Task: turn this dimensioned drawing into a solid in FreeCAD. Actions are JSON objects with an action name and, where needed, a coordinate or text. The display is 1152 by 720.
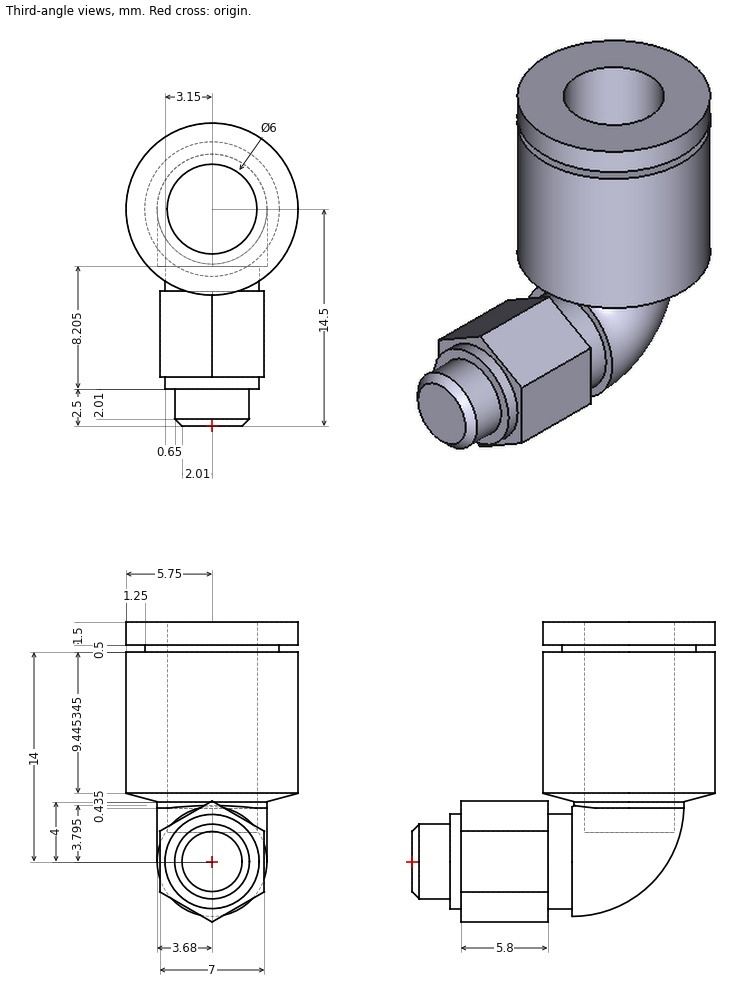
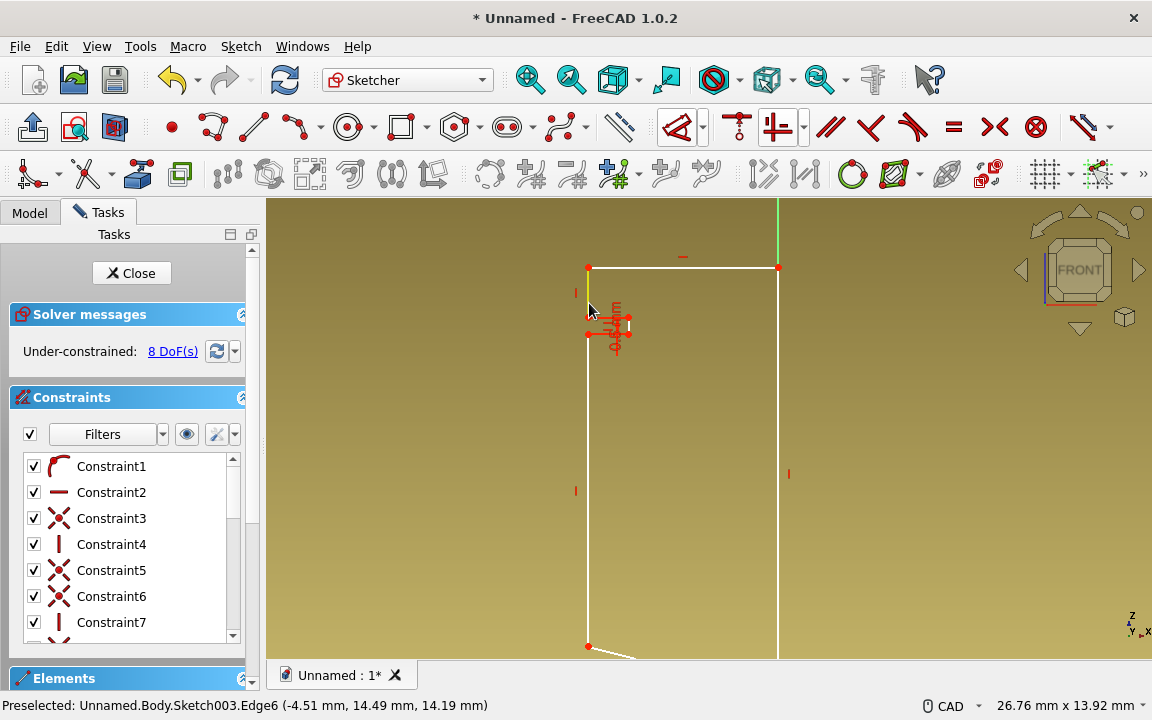
{"action": "left_click", "coordinate": [588, 303]}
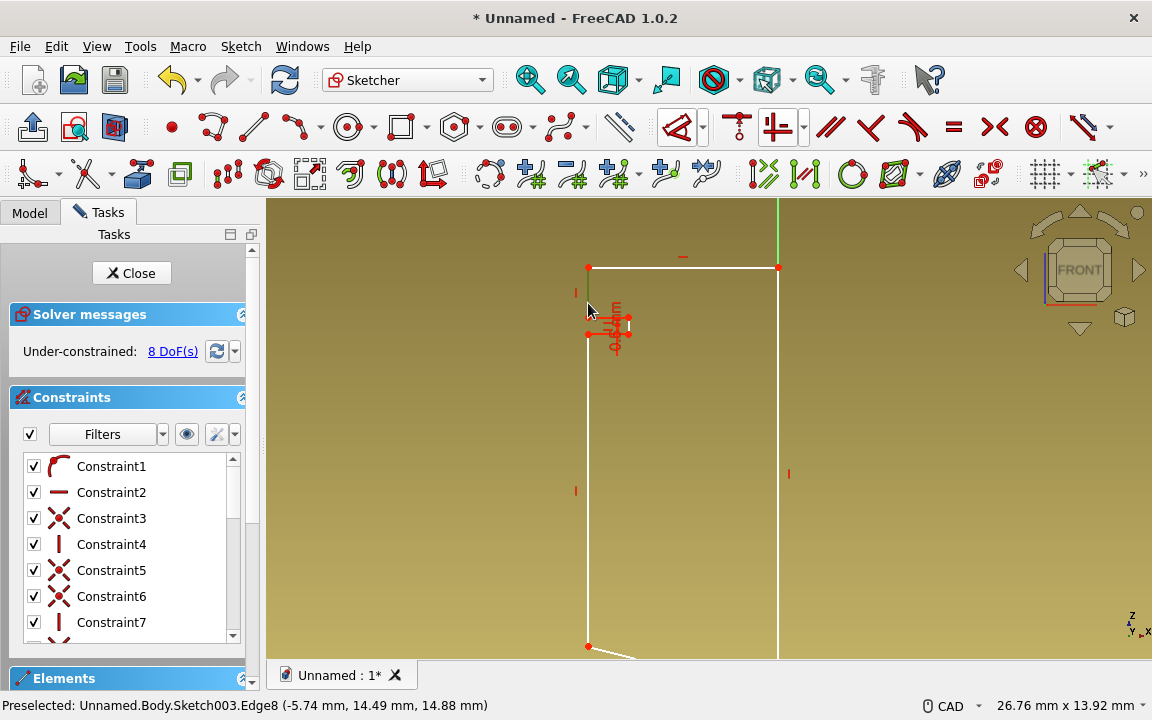
{"action": "key", "text": "i"}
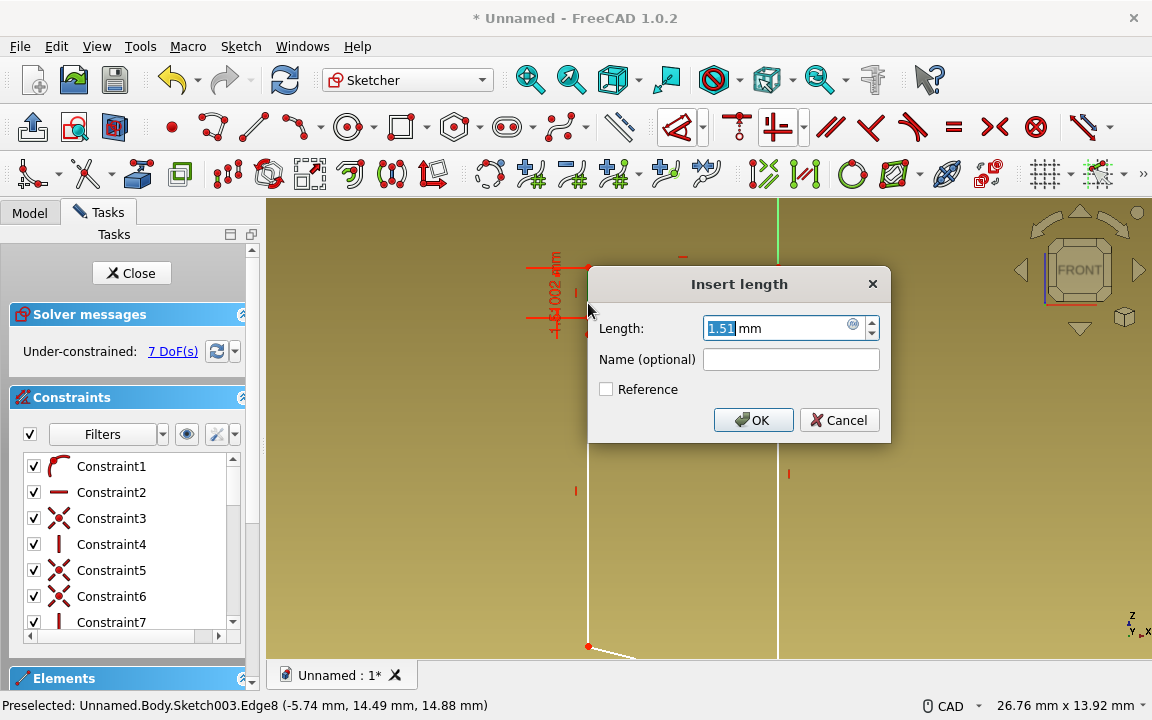
{"action": "type", "text": "1.5"}
{"action": "key", "text": "Return"}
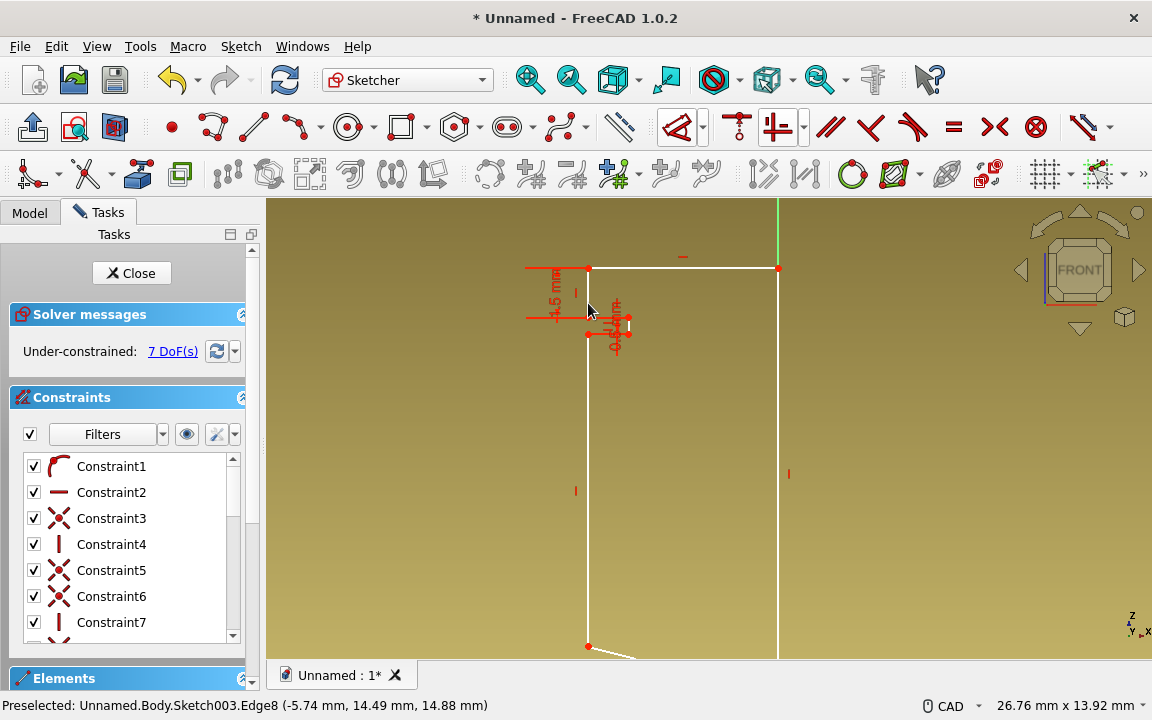
{"action": "left_click", "coordinate": [588, 334]}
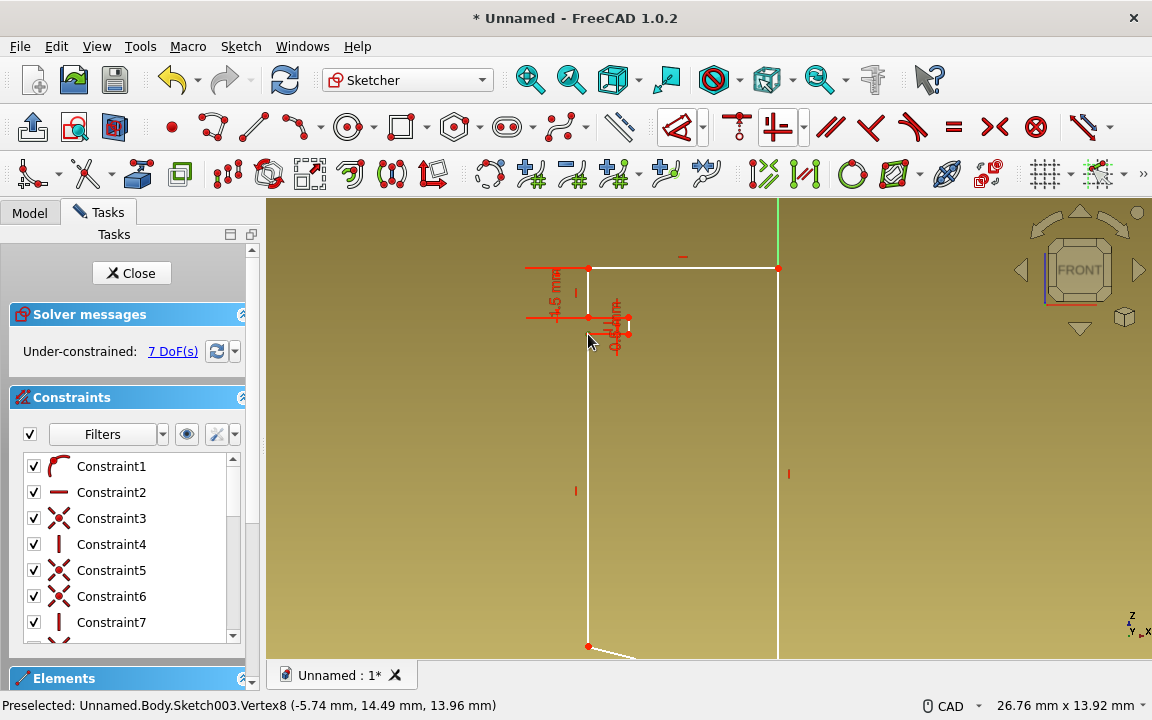
{"action": "left_click", "coordinate": [702, 128]}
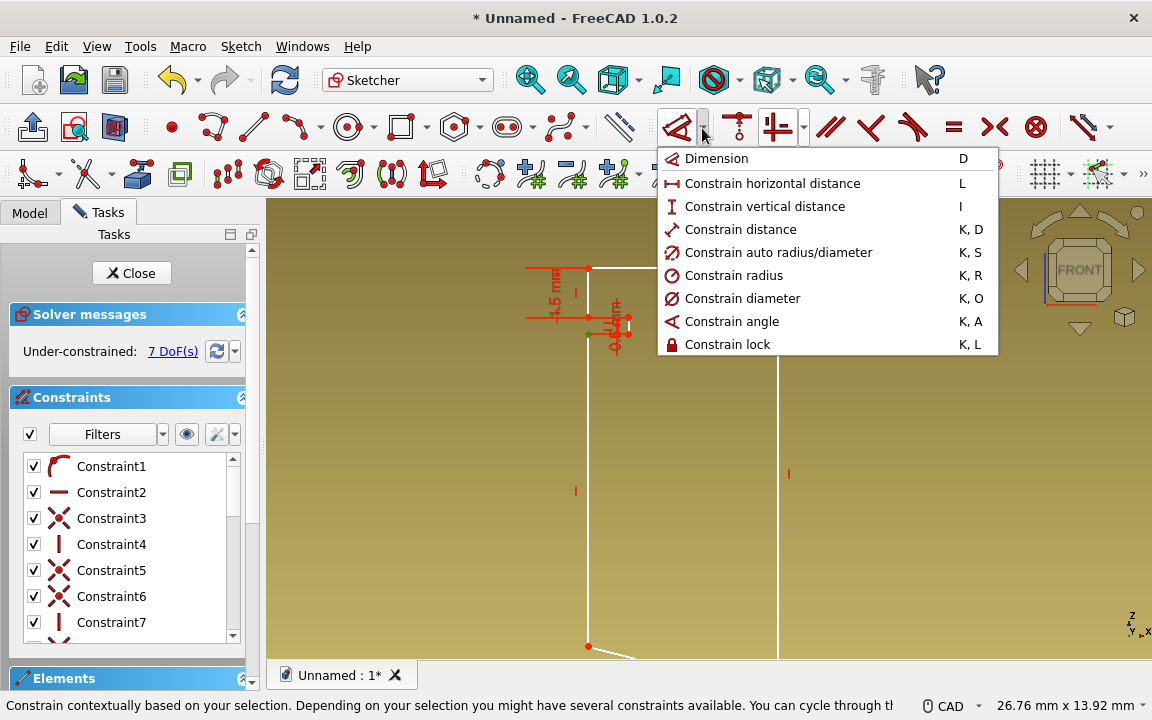
{"action": "left_click", "coordinate": [828, 206]}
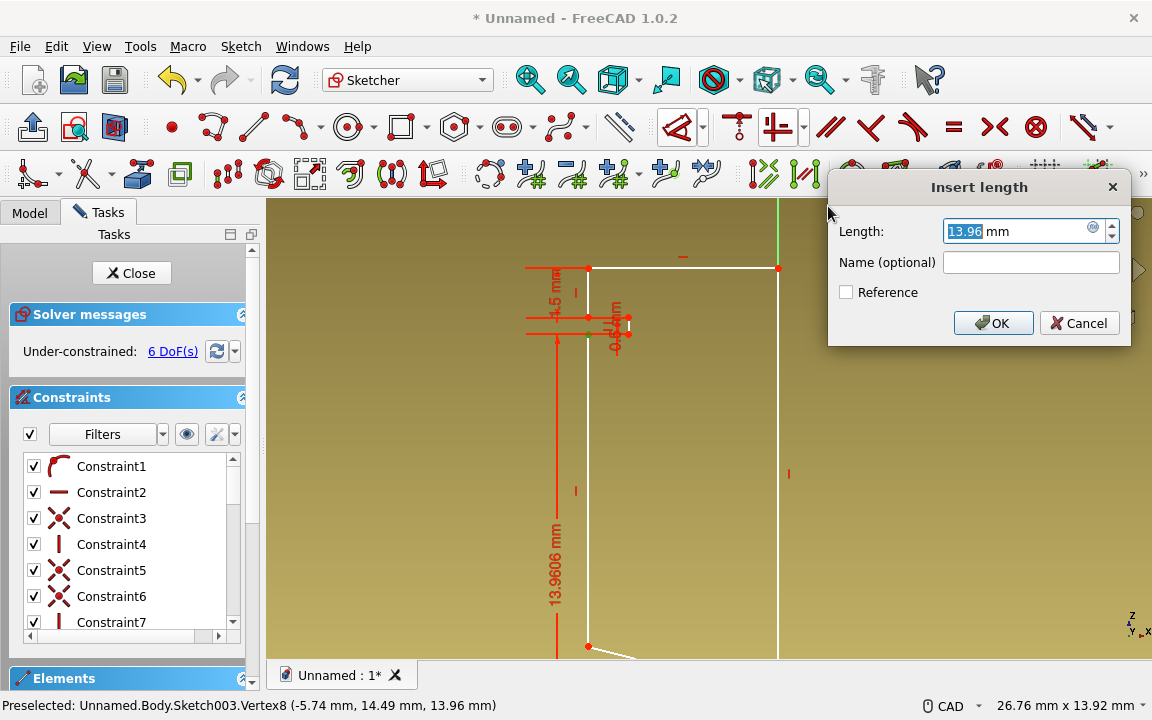
{"action": "type", "text": "14"}
{"action": "key", "text": "Return"}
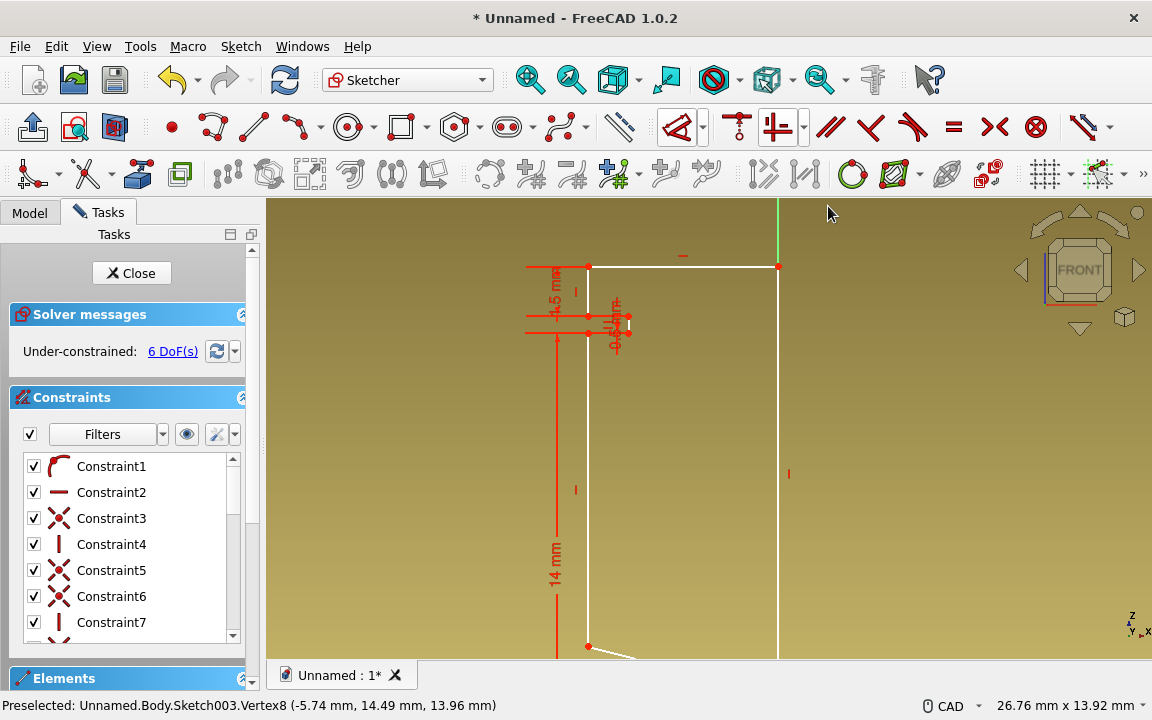
{"action": "scroll", "coordinate": [589, 303], "scroll_direction": "down", "scroll_amount": 3}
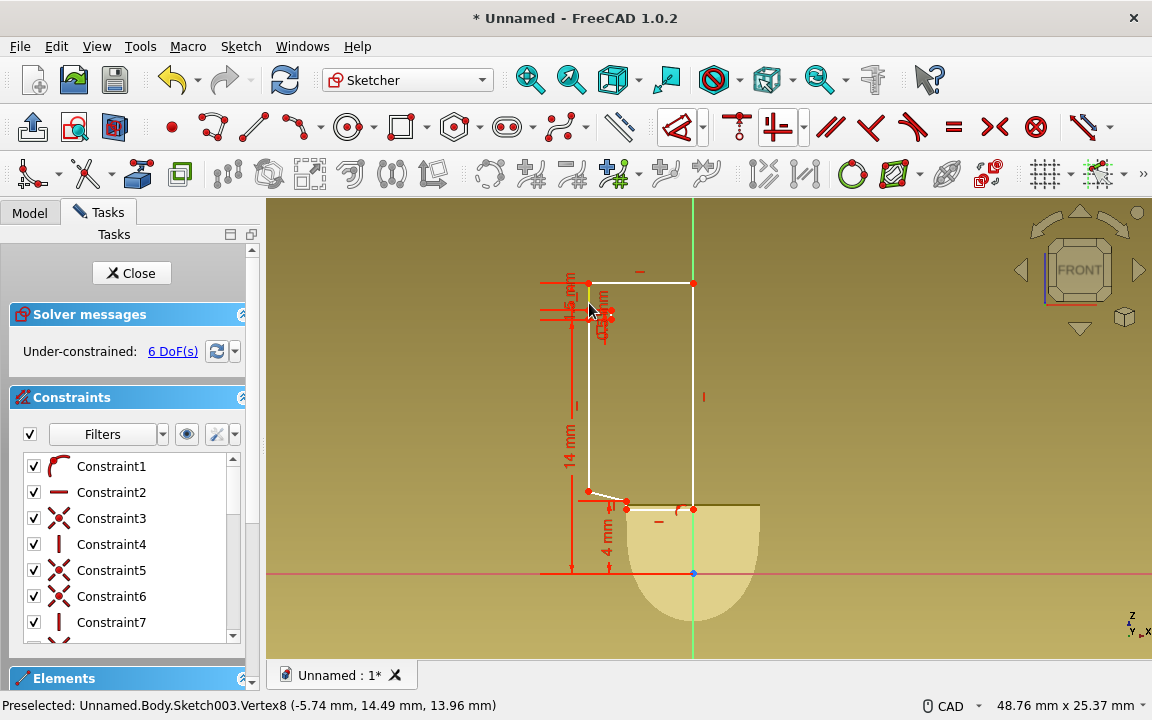
{"action": "left_click", "coordinate": [673, 510]}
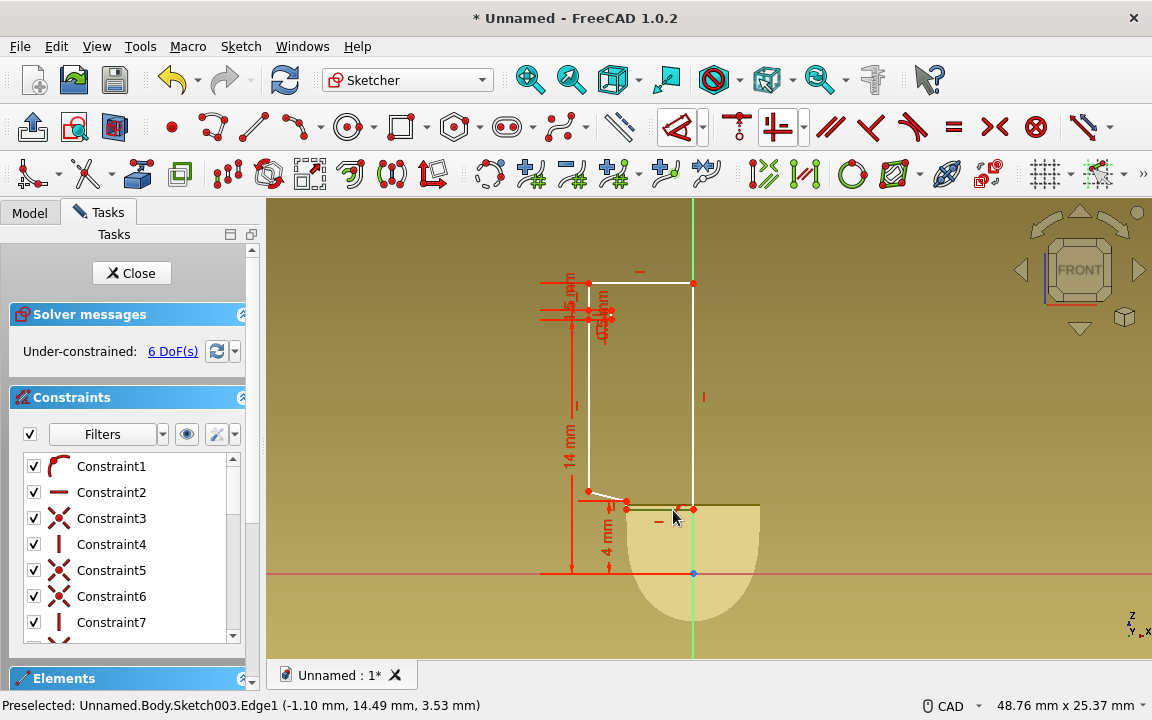
{"action": "left_click", "coordinate": [702, 128]}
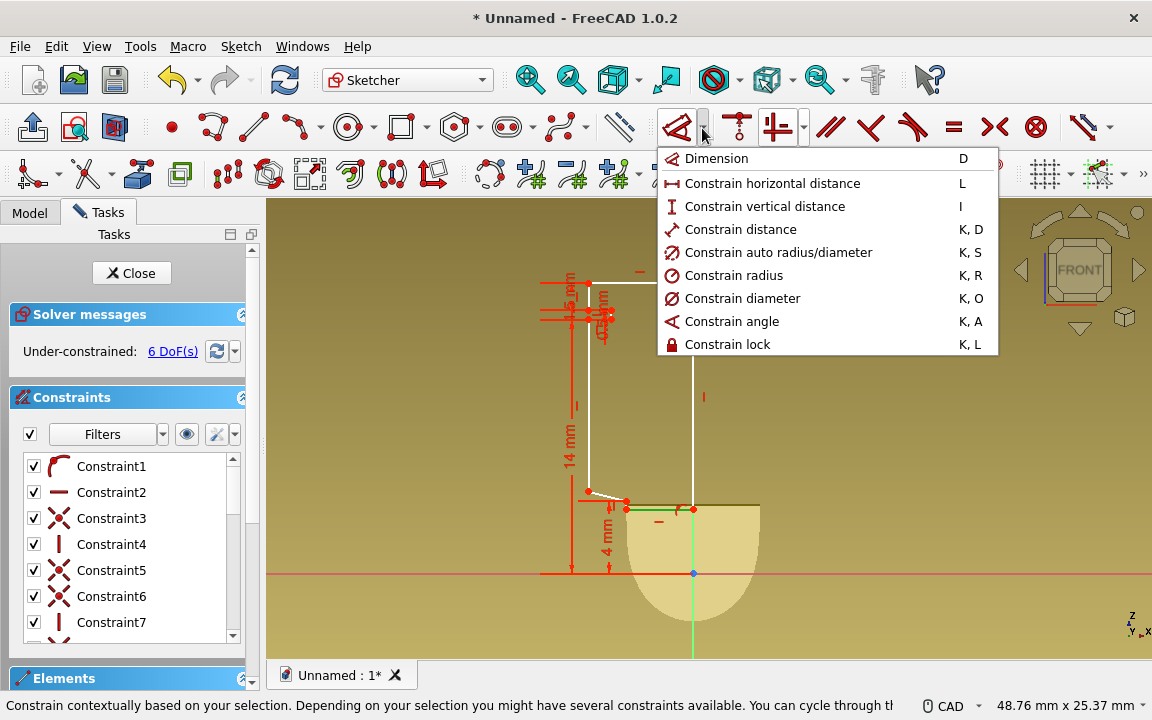
{"action": "left_click", "coordinate": [828, 184]}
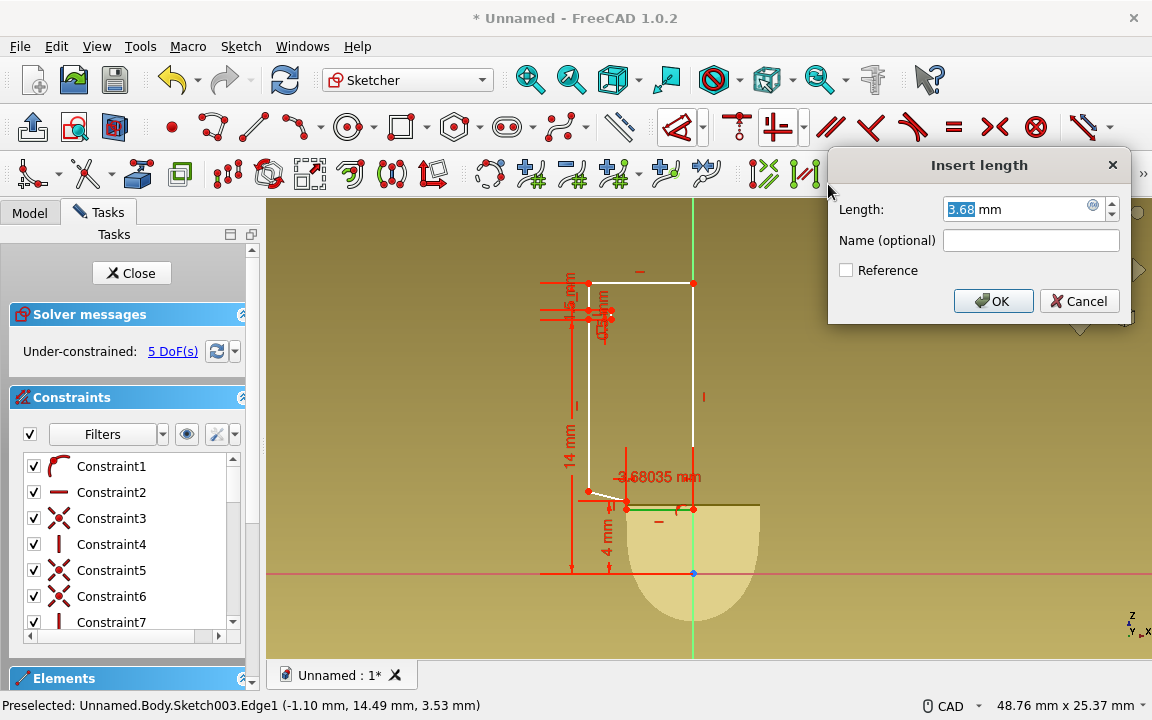
{"action": "type", "text": "3.68"}
{"action": "key", "text": "Return"}